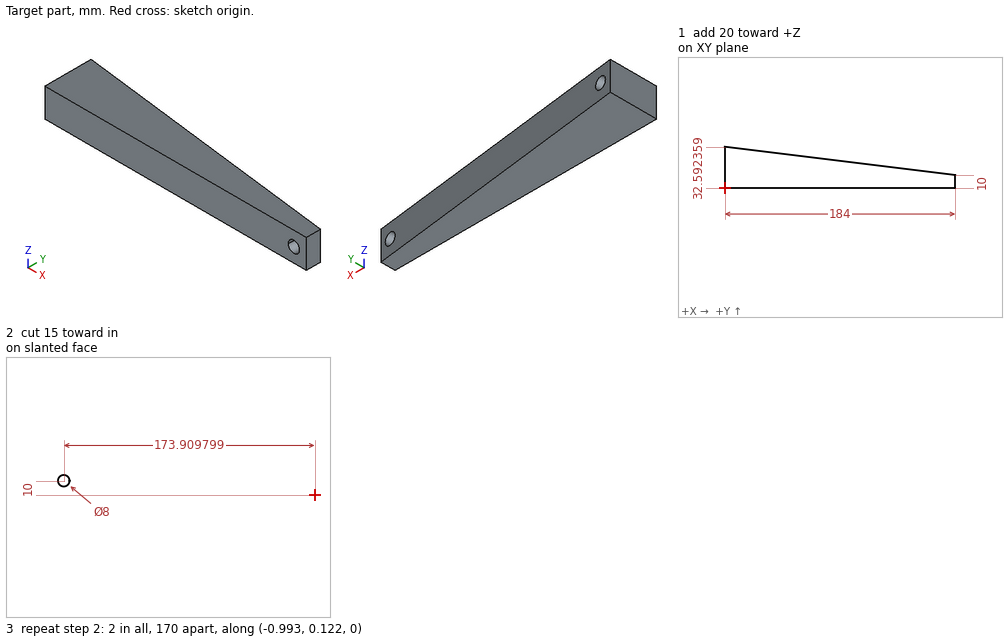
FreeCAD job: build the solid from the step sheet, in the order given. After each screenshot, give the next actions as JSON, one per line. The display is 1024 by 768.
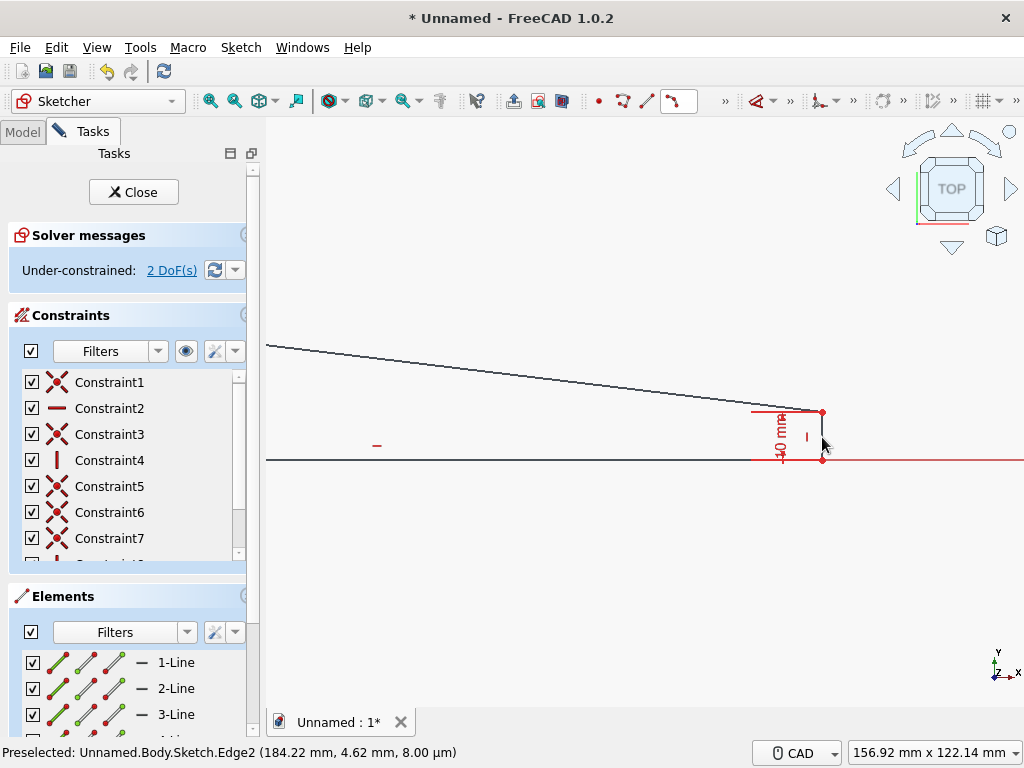
{"action": "left_click", "coordinate": [555, 460]}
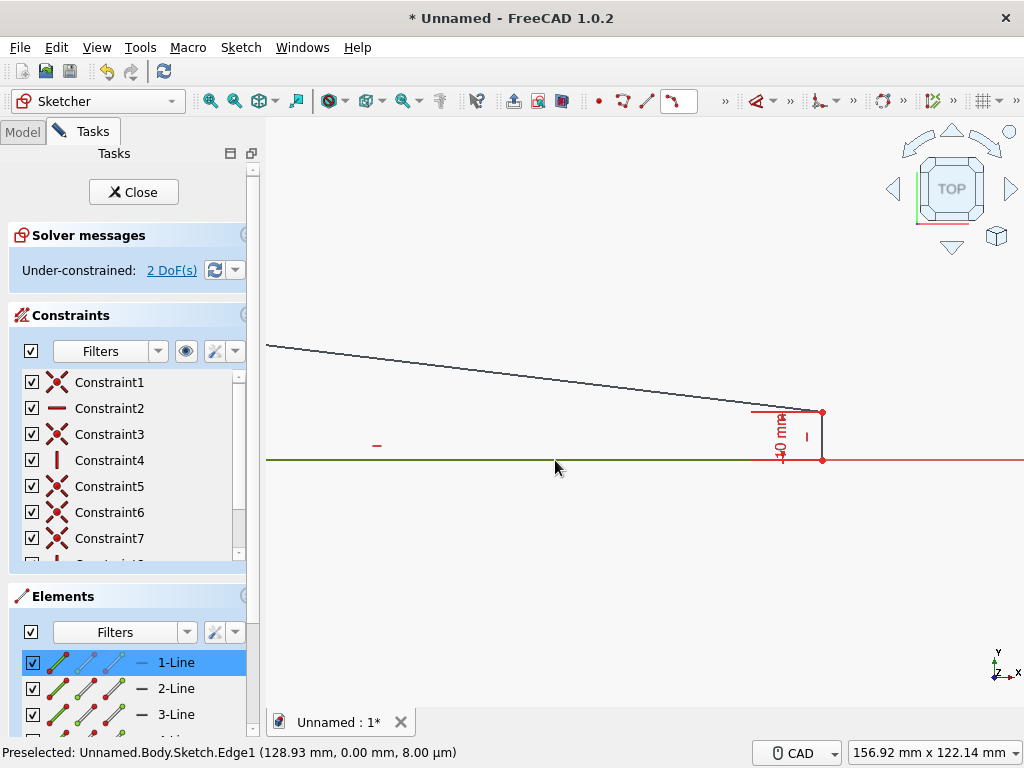
{"action": "left_click", "coordinate": [776, 102]}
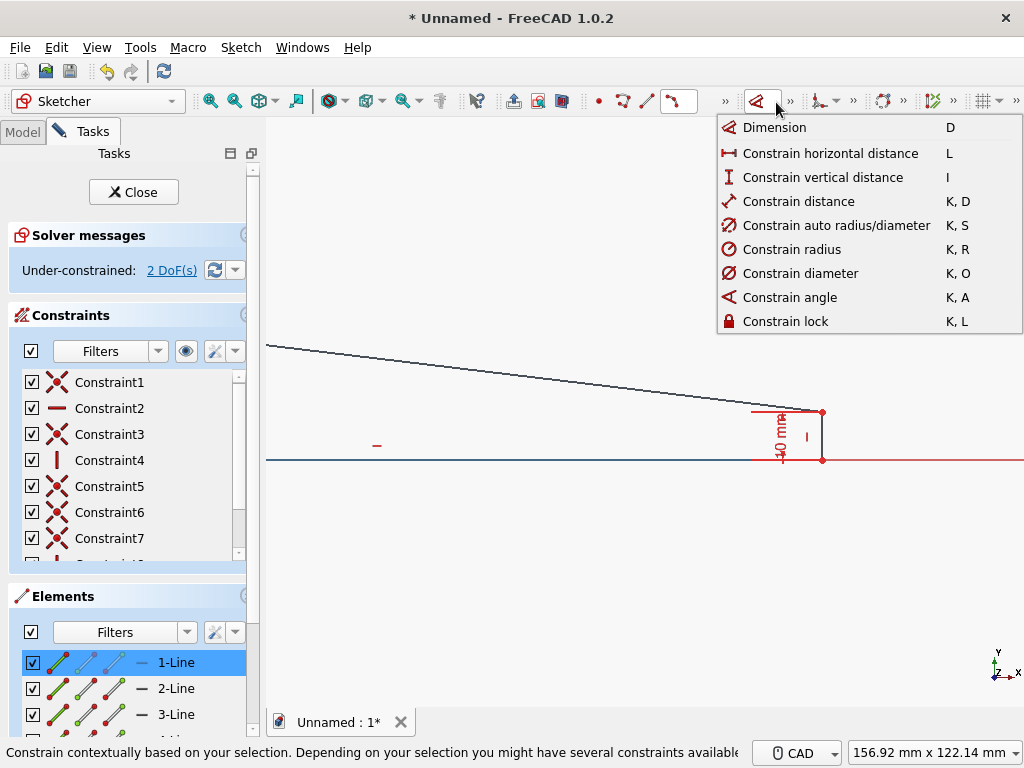
{"action": "left_click", "coordinate": [870, 153]}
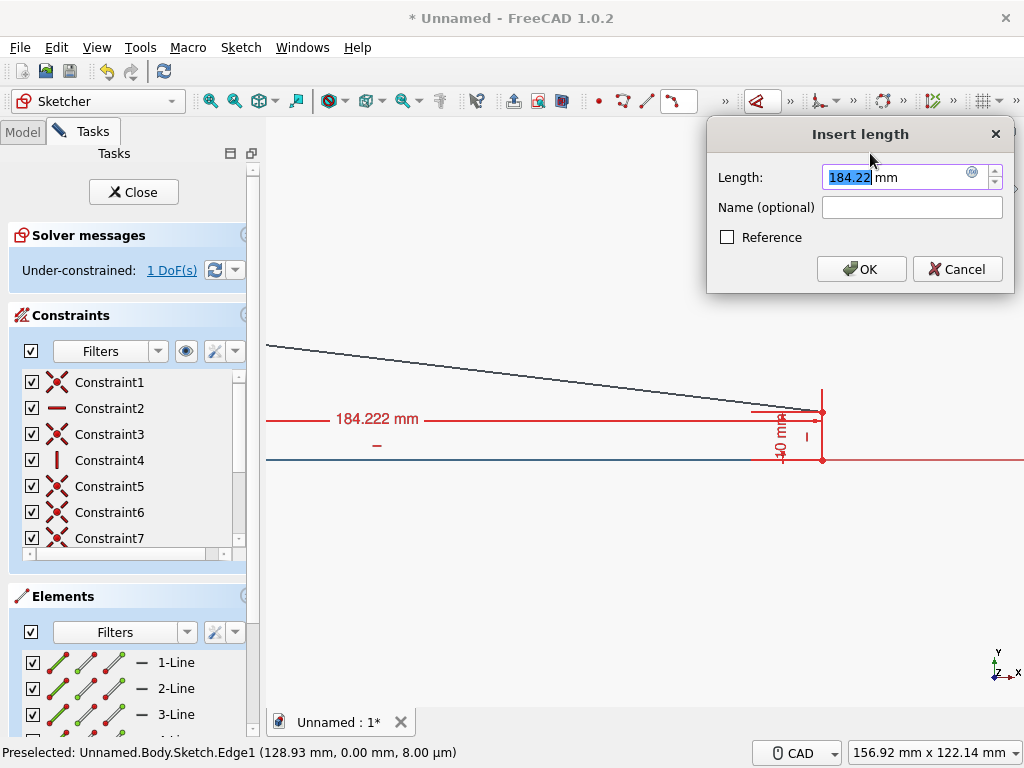
{"action": "type", "text": "184"}
{"action": "key", "text": "Return"}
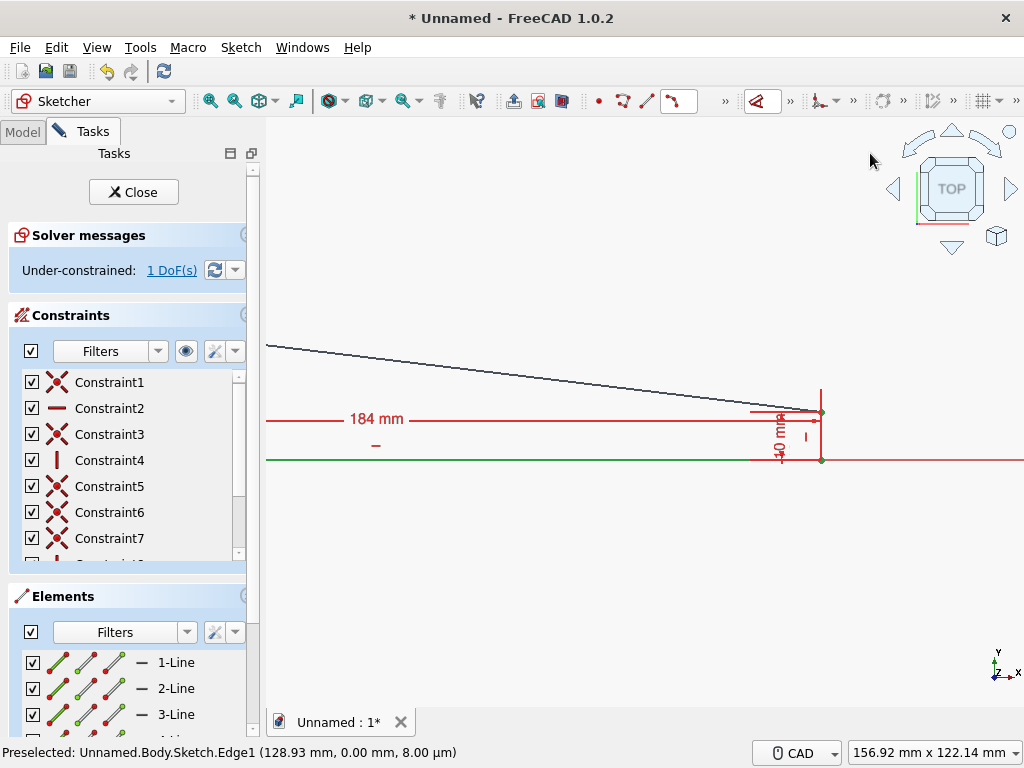
{"action": "scroll", "coordinate": [740, 437], "scroll_direction": "down", "scroll_amount": 4}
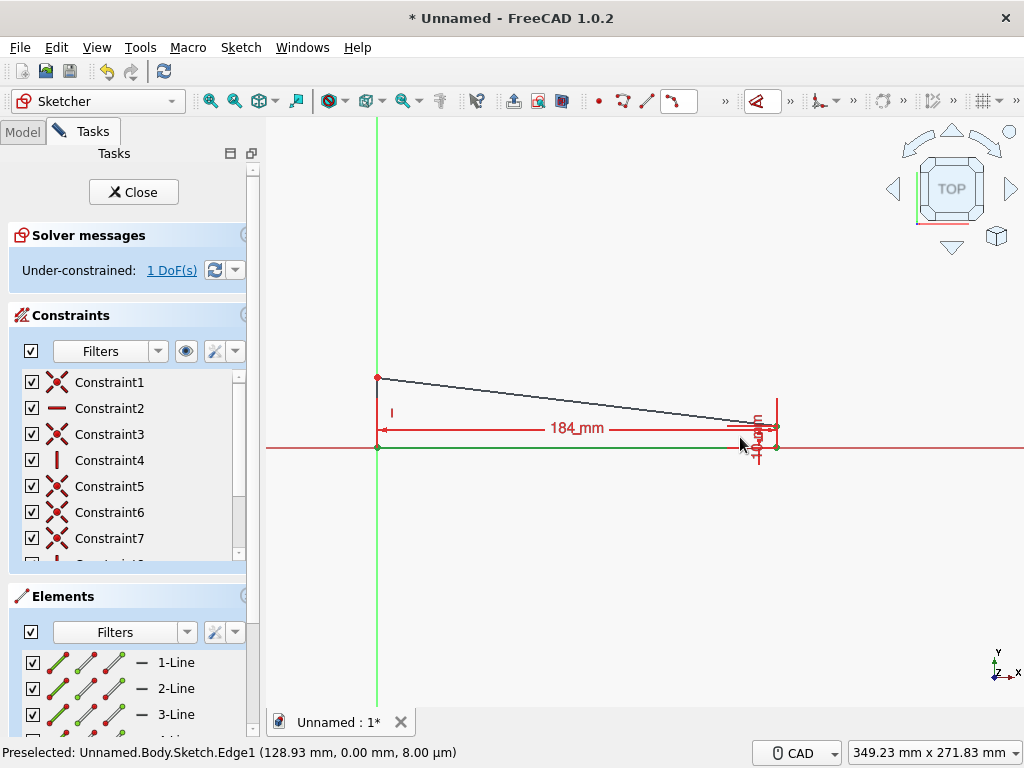
{"action": "left_click", "coordinate": [377, 399]}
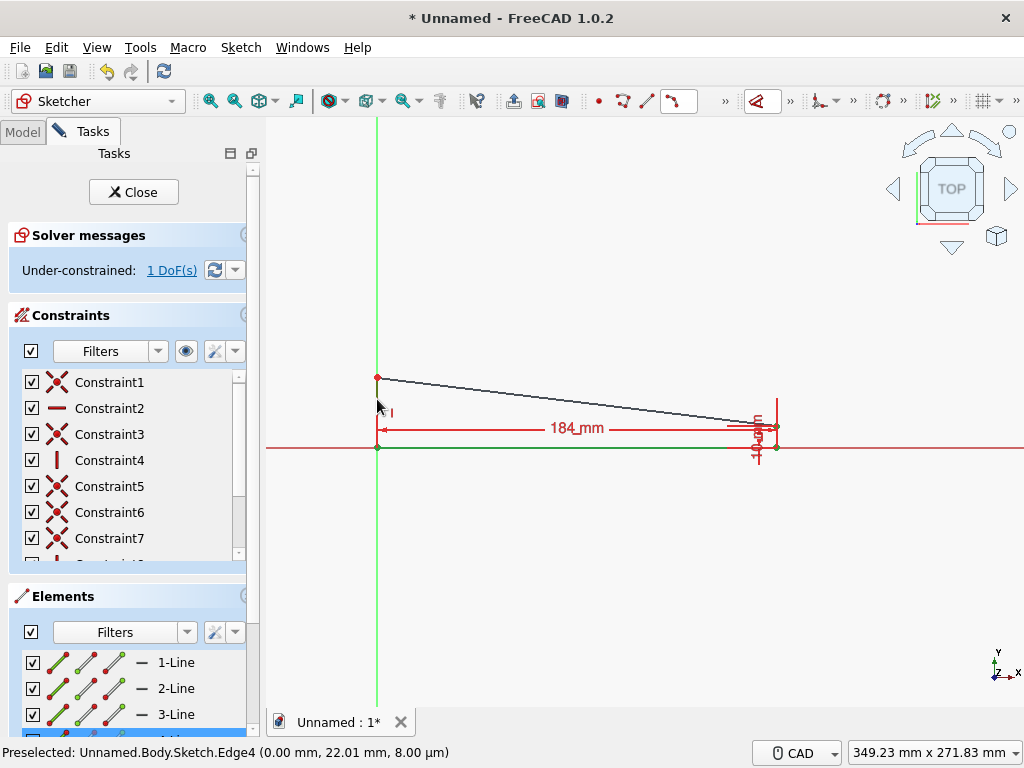
{"action": "key", "text": "i"}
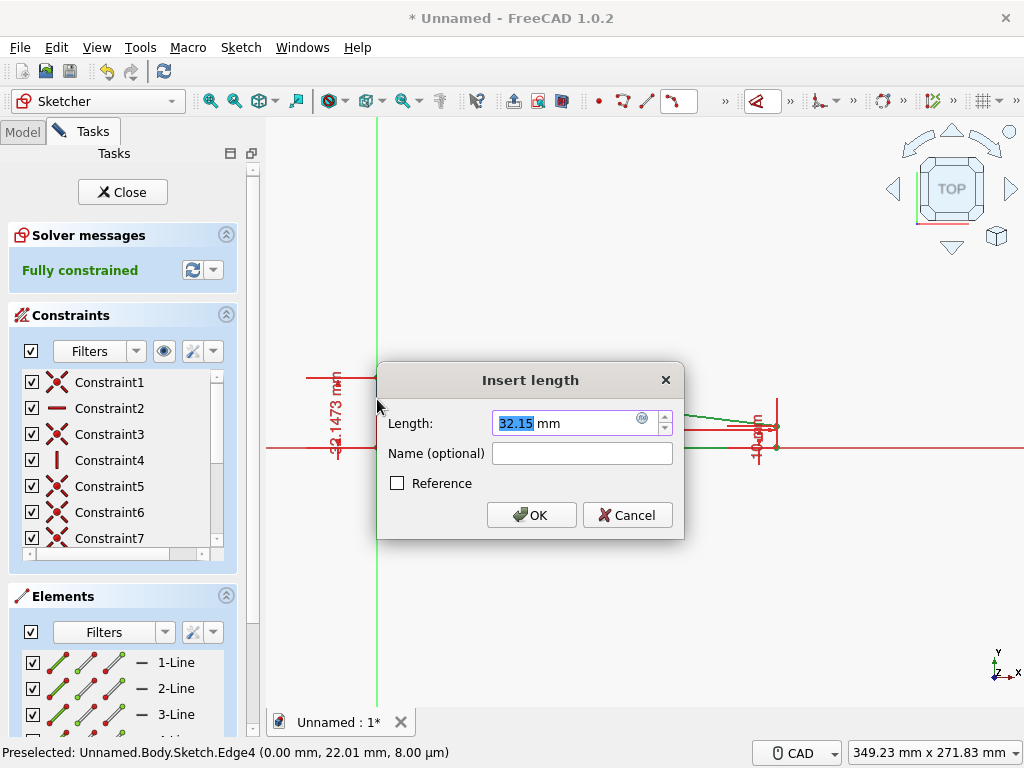
{"action": "type", "text": "32.592359"}
{"action": "key", "text": "Return"}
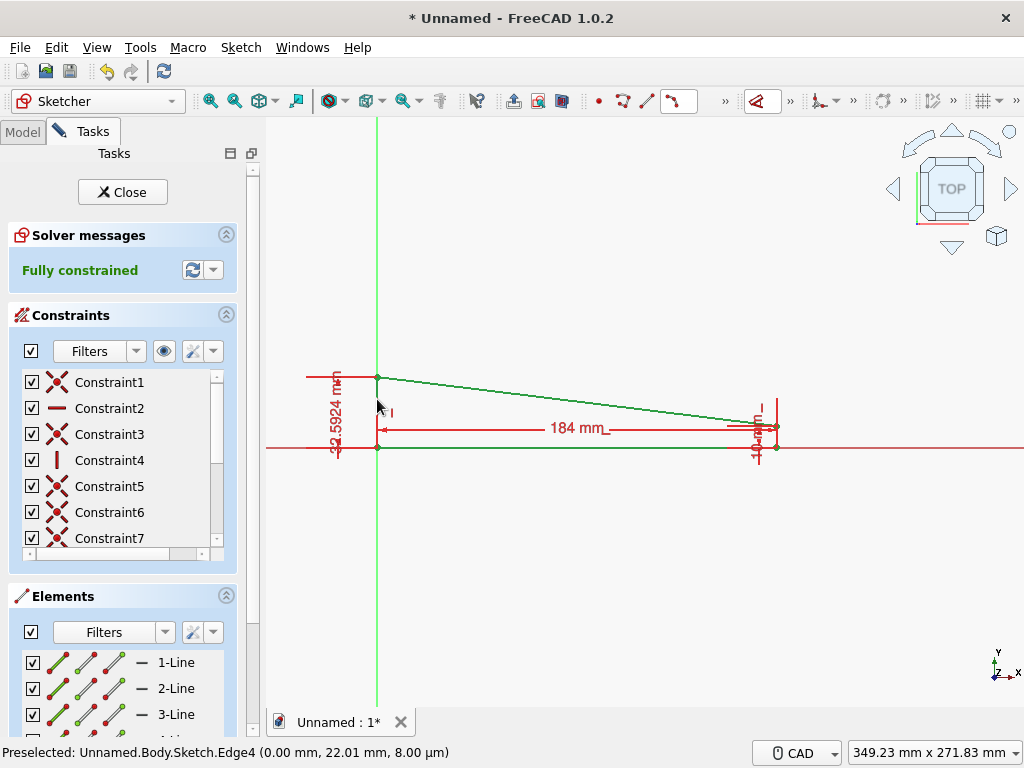
{"action": "left_click", "coordinate": [123, 192]}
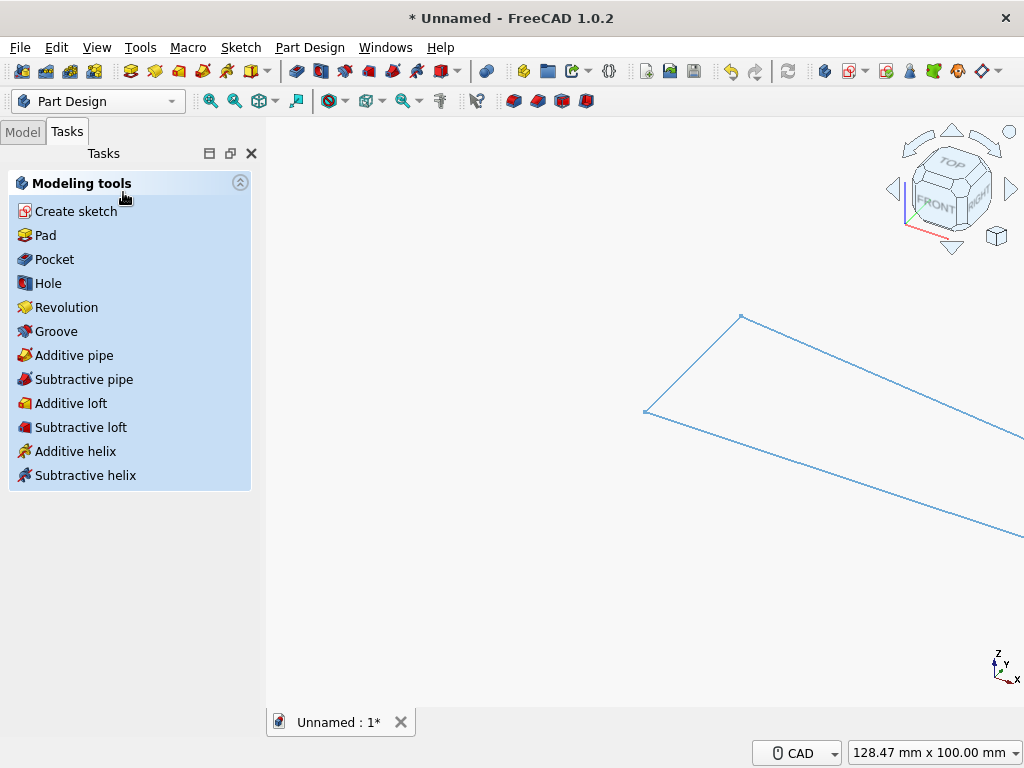
{"action": "left_click", "coordinate": [132, 72]}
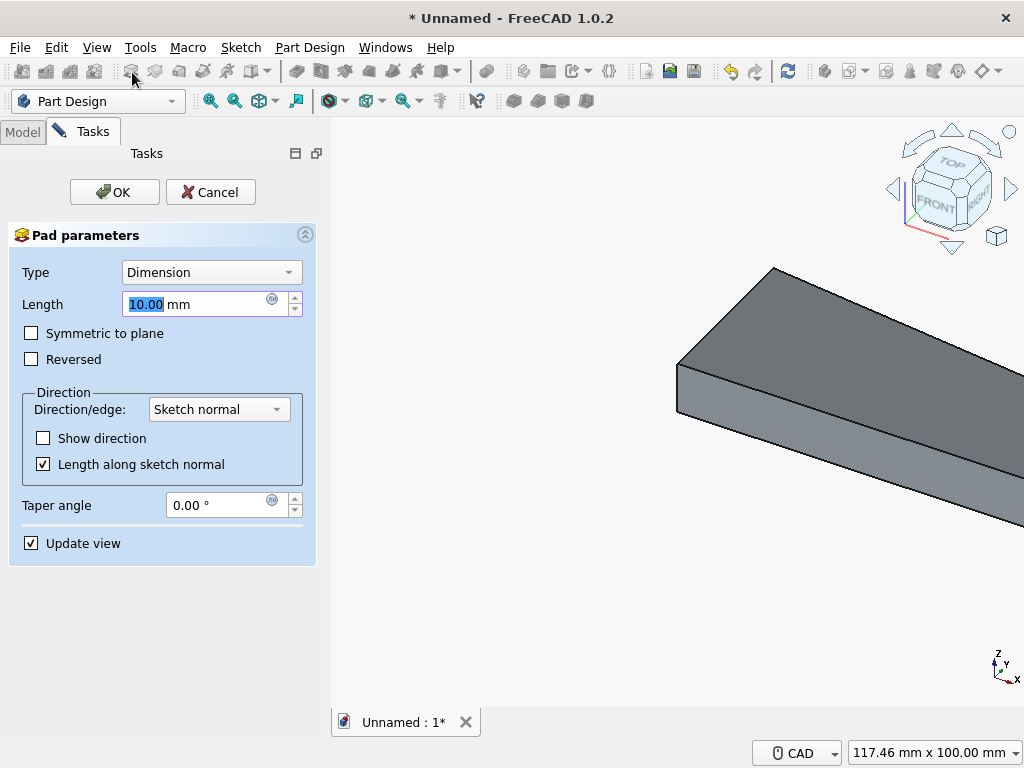
{"action": "type", "text": "20"}
{"action": "key", "text": "Tab"}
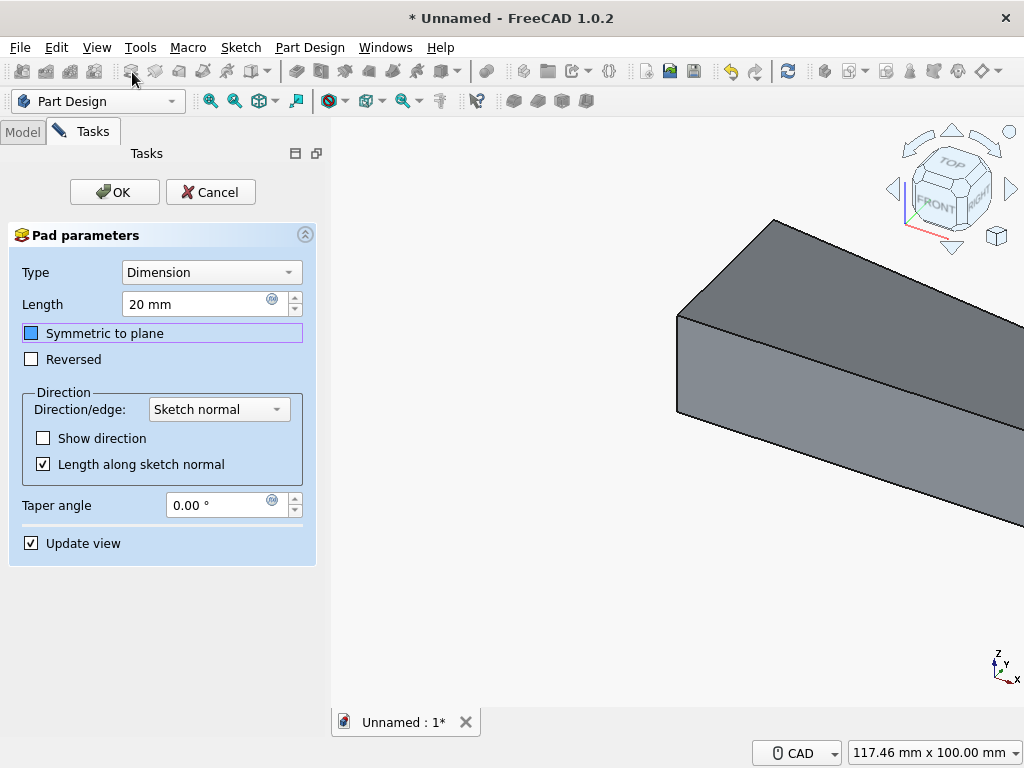
{"action": "left_click", "coordinate": [115, 192]}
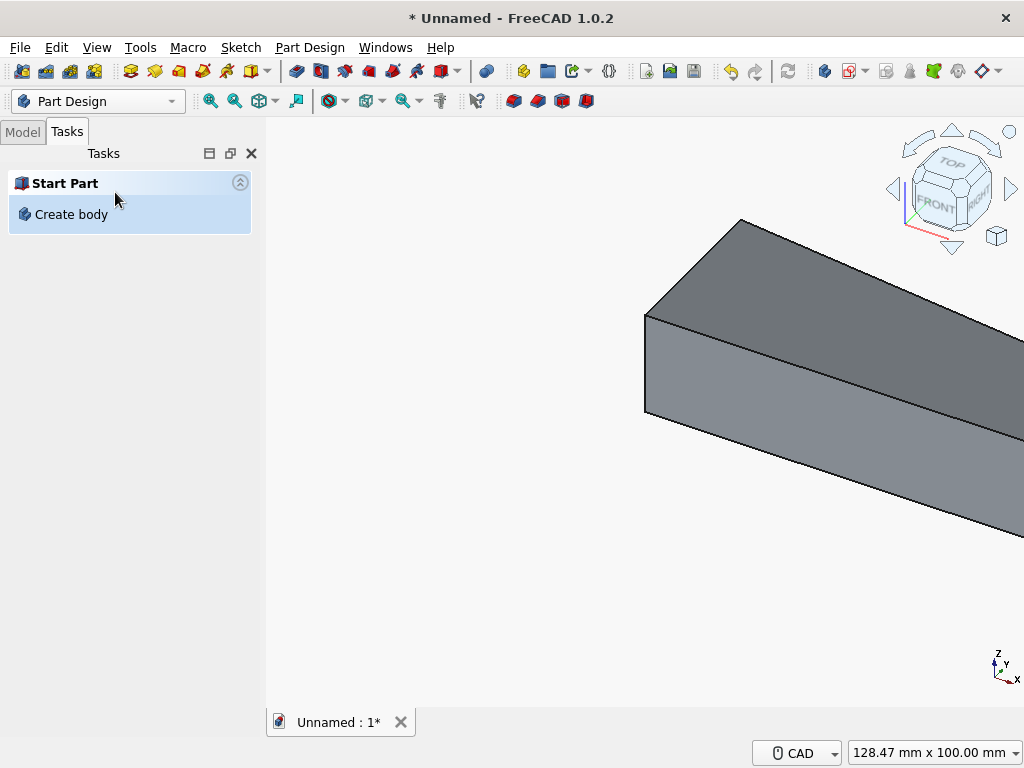
{"action": "left_click", "coordinate": [212, 102]}